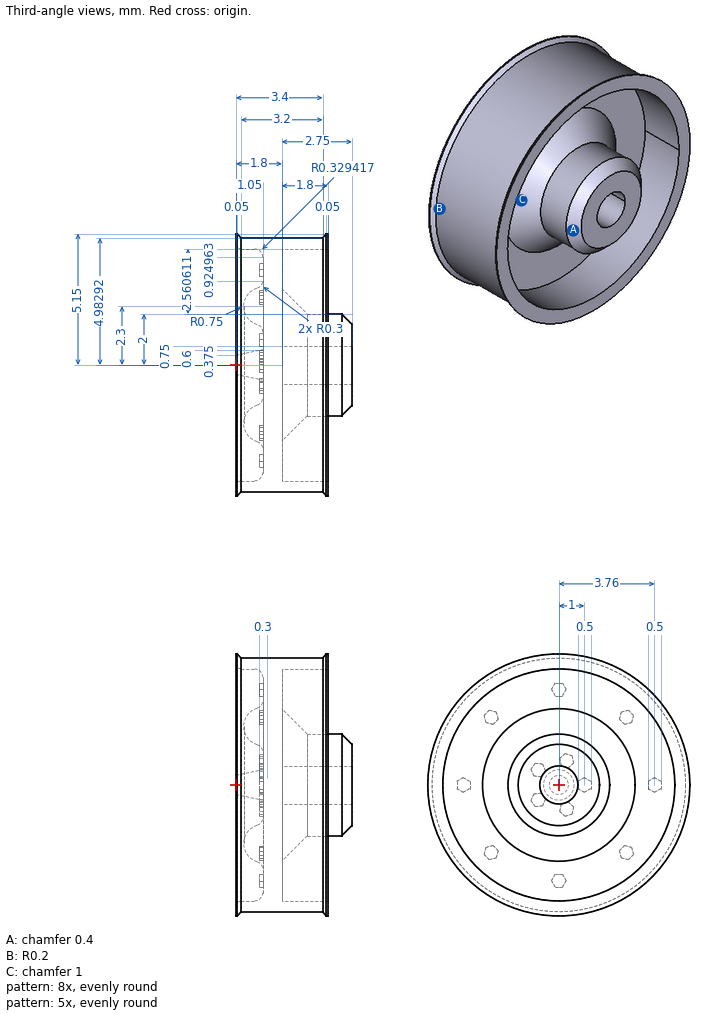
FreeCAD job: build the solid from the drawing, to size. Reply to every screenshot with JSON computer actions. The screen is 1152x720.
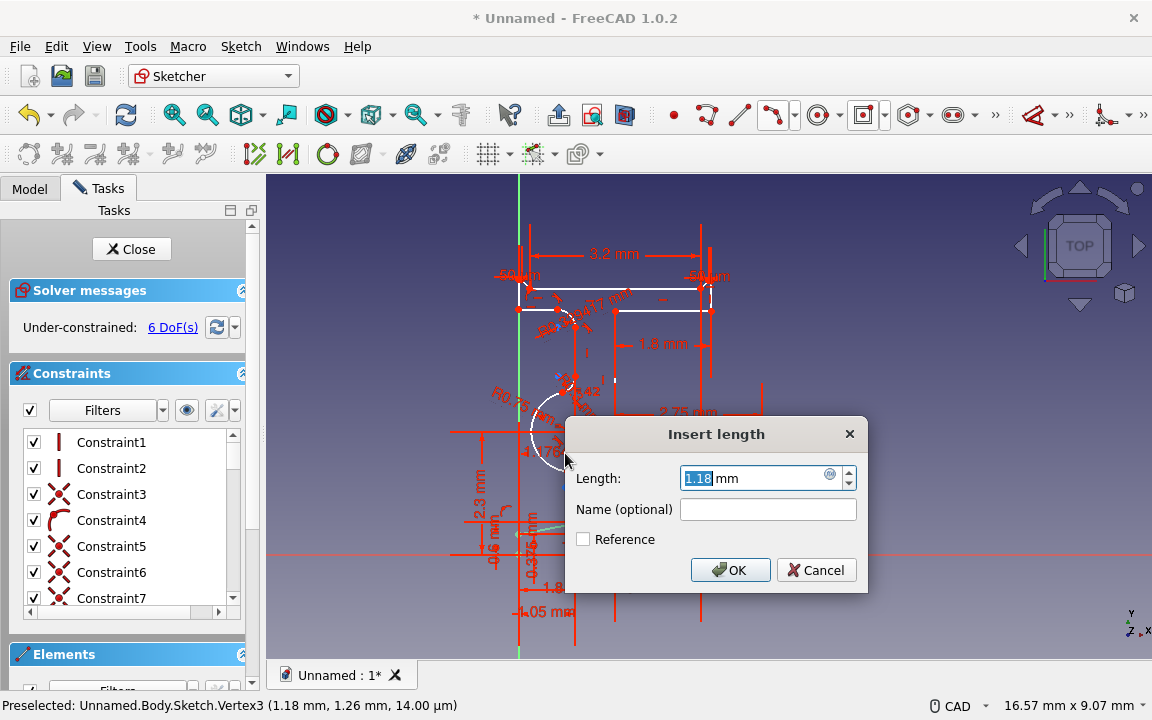
{"action": "type", "text": "1.05"}
{"action": "key", "text": "Return"}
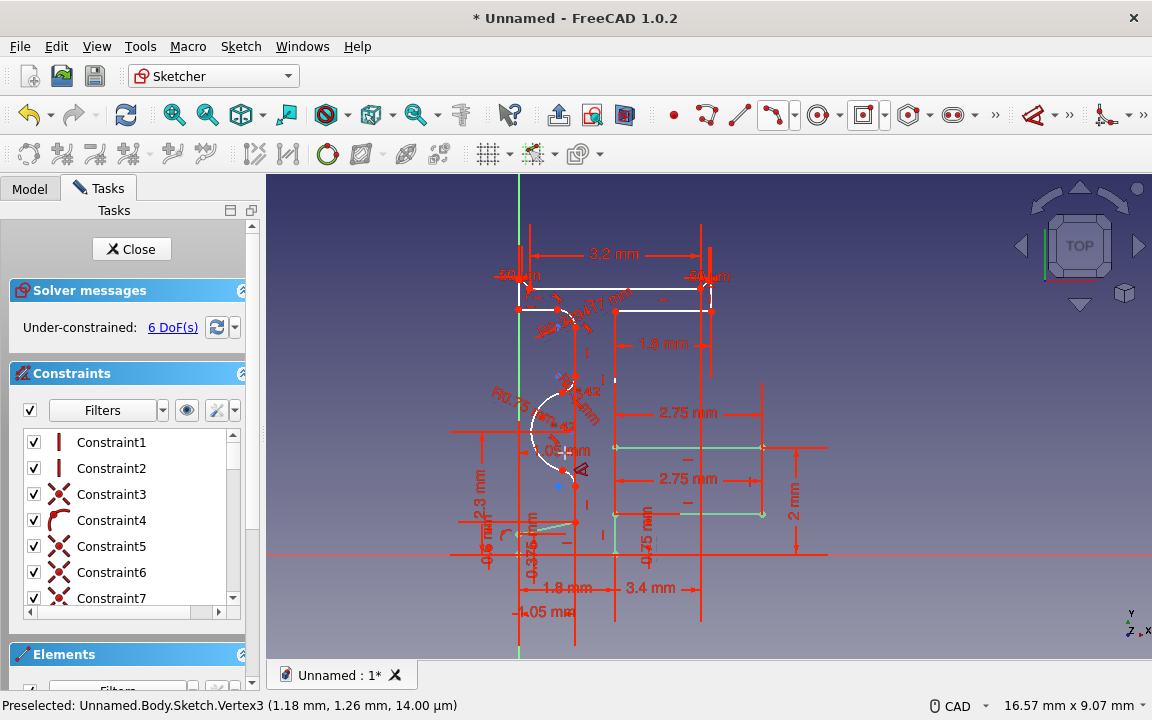
{"action": "scroll", "coordinate": [711, 280], "scroll_direction": "up", "scroll_amount": 8}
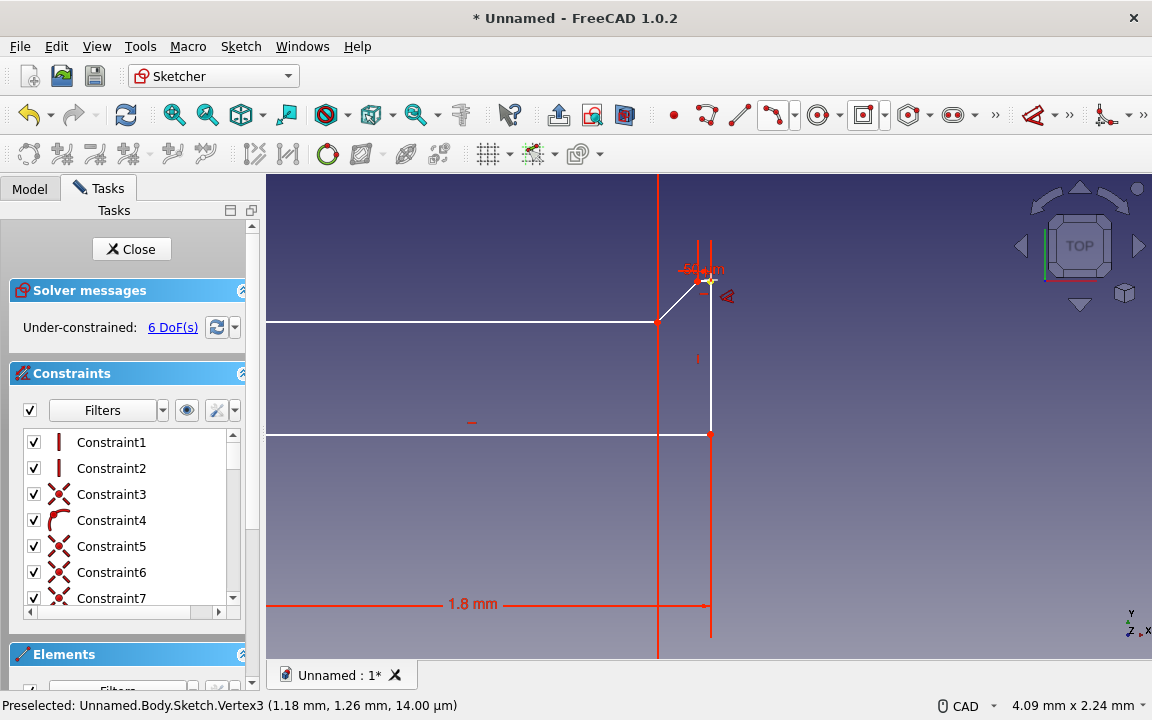
{"action": "left_click", "coordinate": [711, 281]}
{"action": "left_click", "coordinate": [745, 456]}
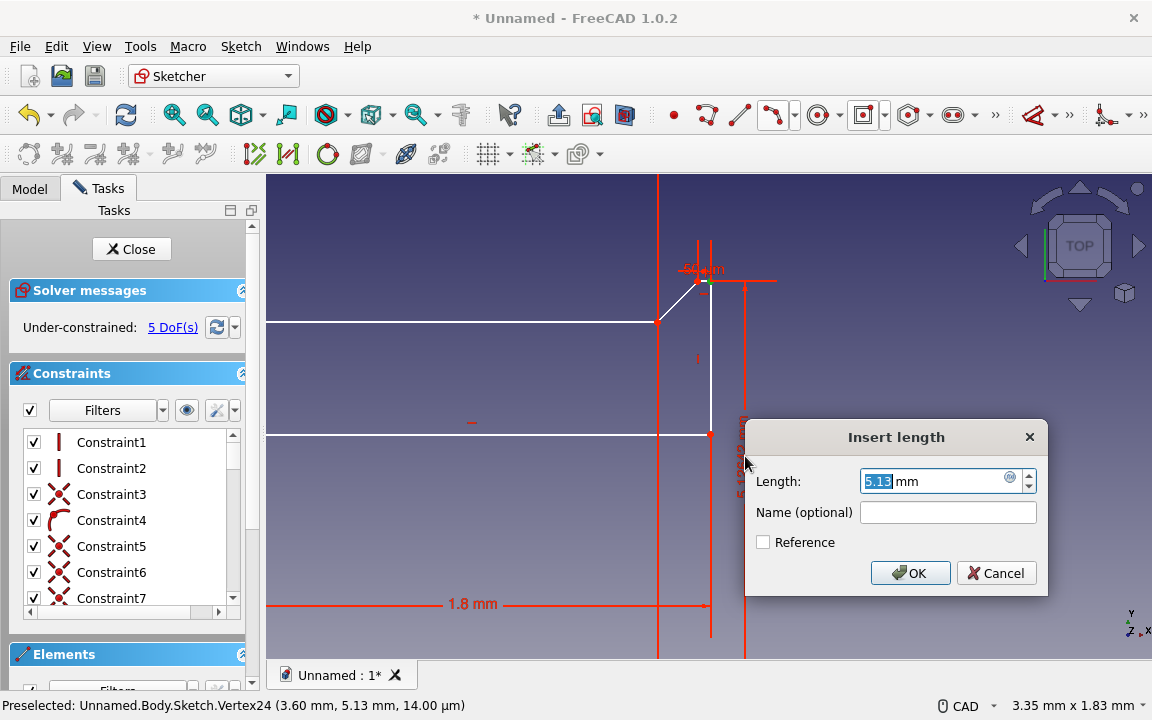
{"action": "type", "text": "5.15"}
{"action": "key", "text": "Return"}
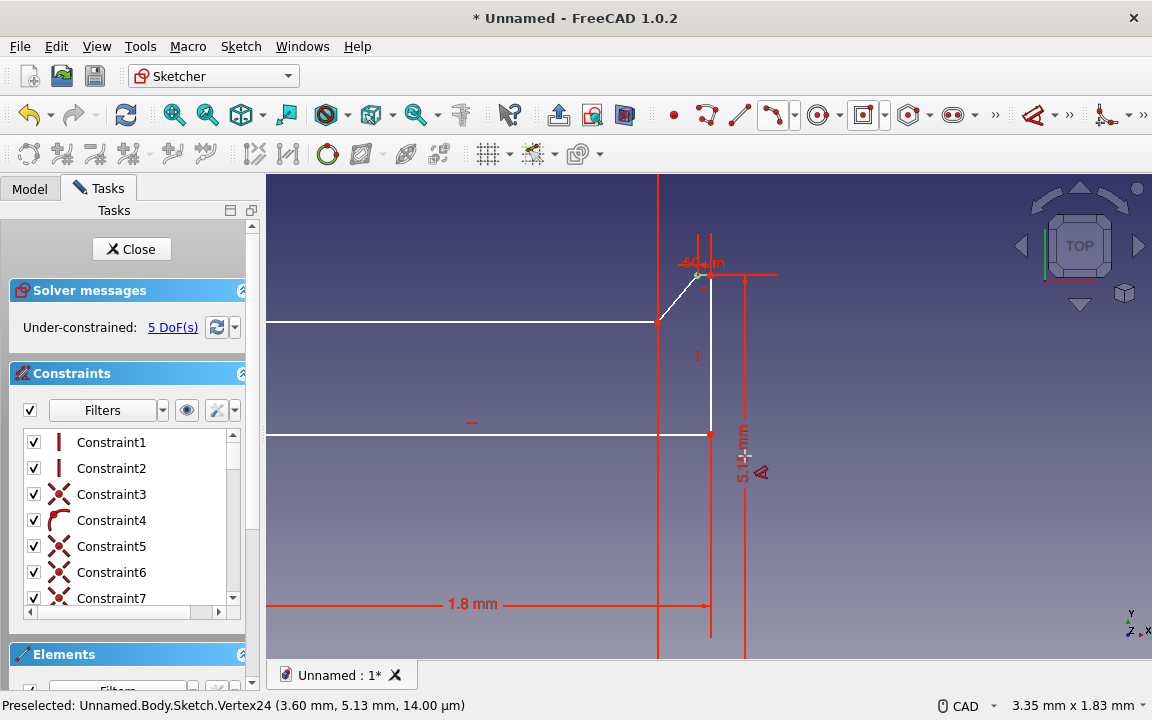
{"action": "scroll", "coordinate": [711, 280], "scroll_direction": "down", "scroll_amount": 8}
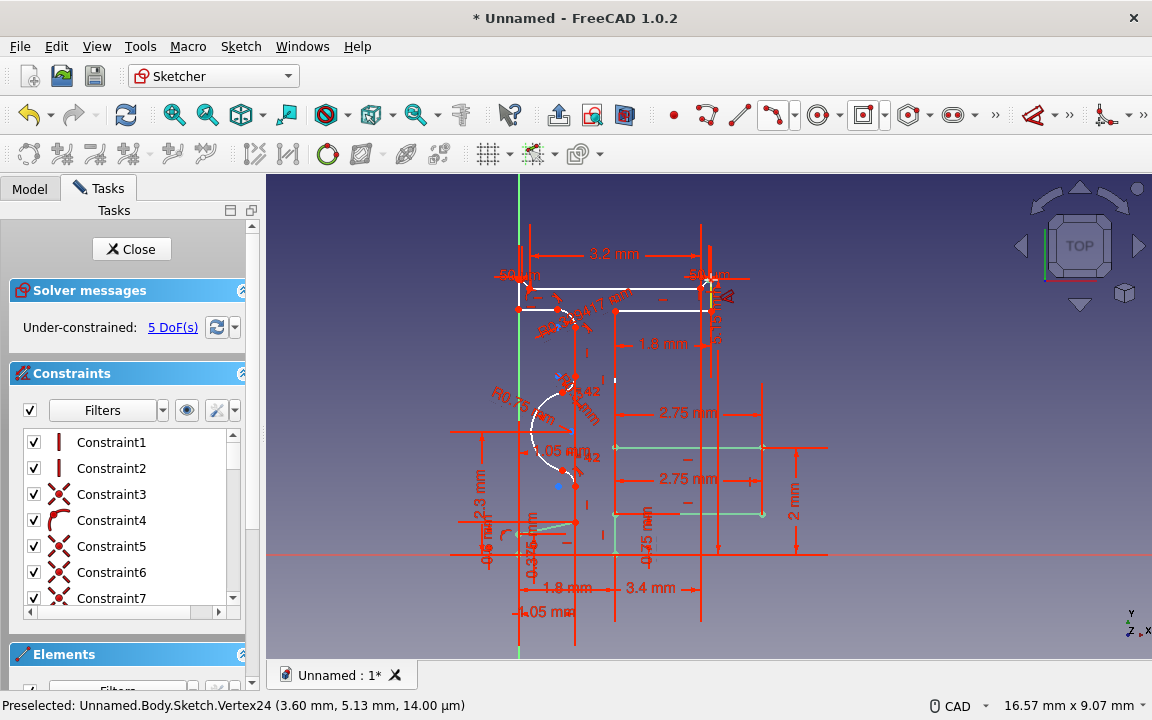
{"action": "scroll", "coordinate": [522, 279], "scroll_direction": "up", "scroll_amount": 8}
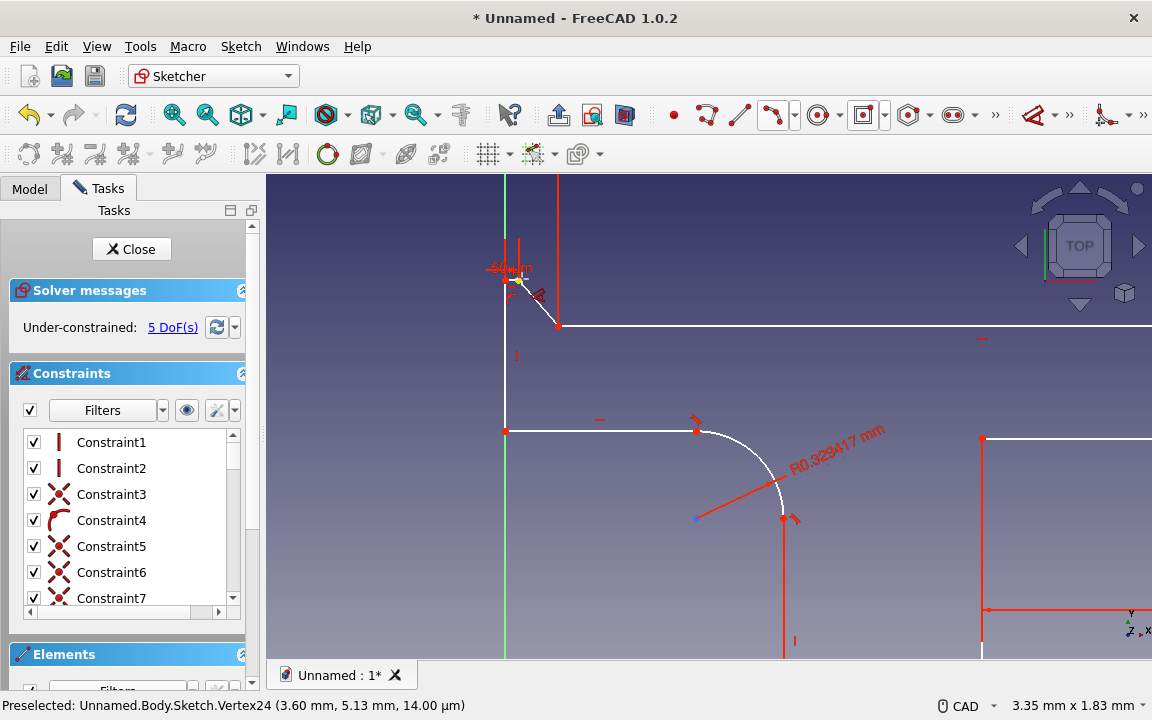
{"action": "left_click", "coordinate": [519, 280]}
{"action": "left_click", "coordinate": [471, 456]}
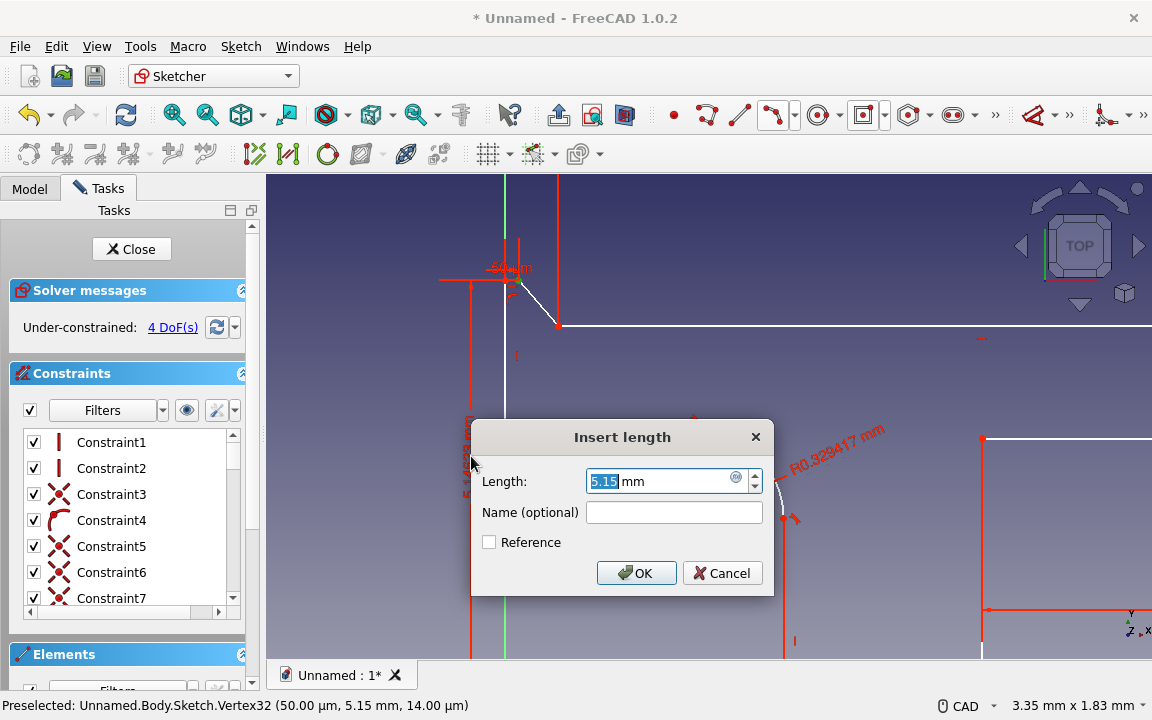
{"action": "type", "text": "5.15"}
{"action": "key", "text": "Return"}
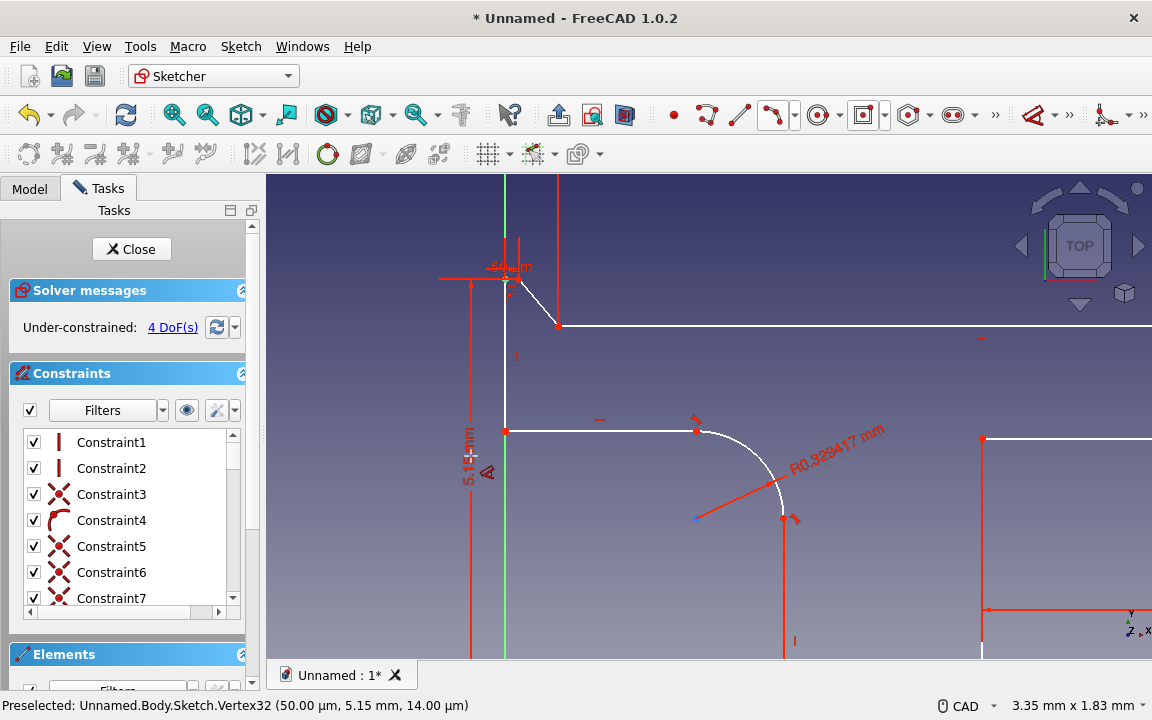
{"action": "scroll", "coordinate": [522, 279], "scroll_direction": "down", "scroll_amount": 8}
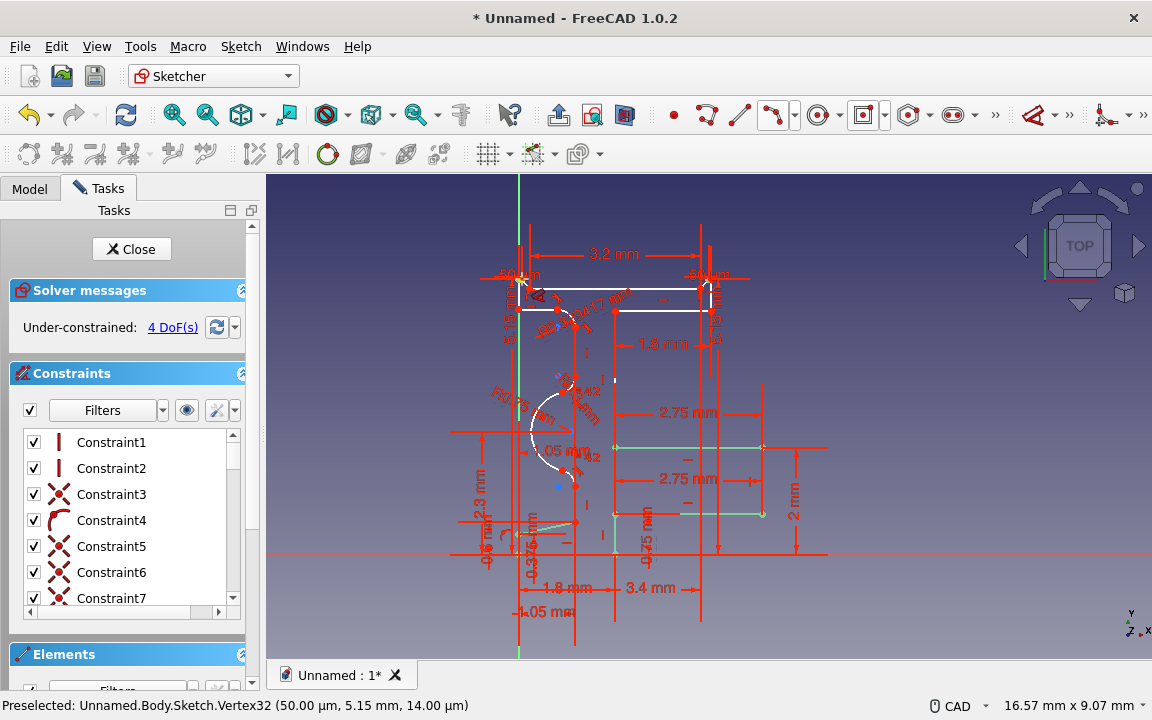
{"action": "left_click", "coordinate": [571, 432]}
{"action": "left_click", "coordinate": [545, 374]}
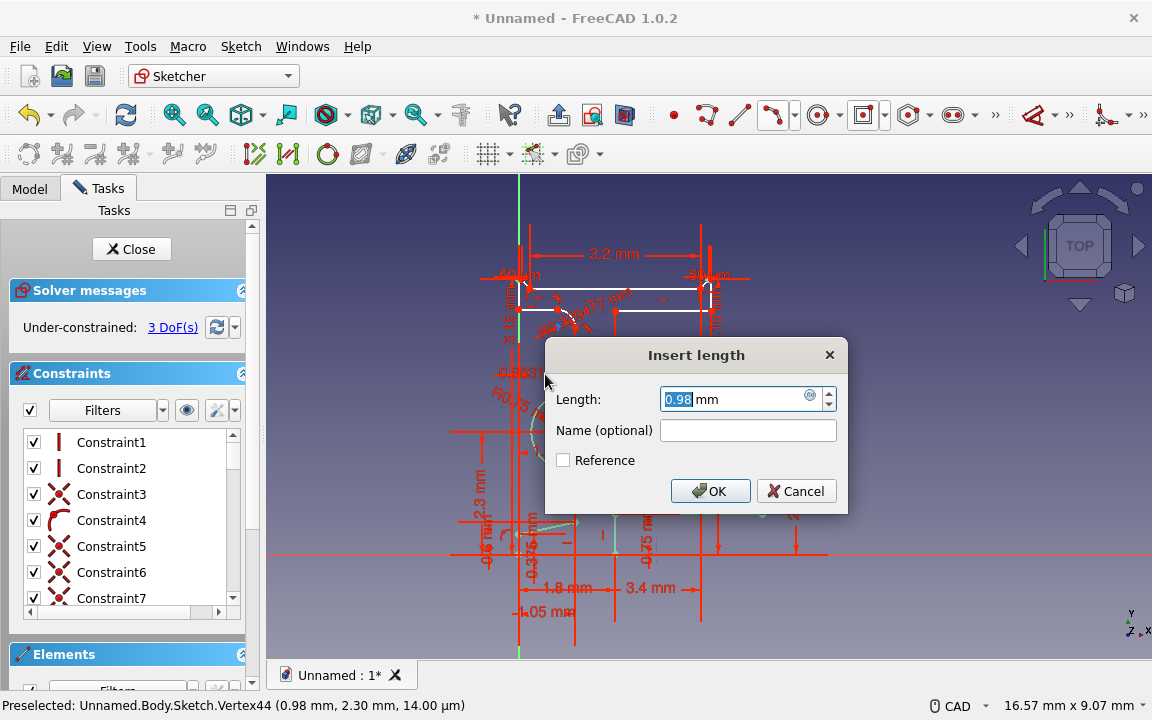
{"action": "type", "text": "1.05"}
{"action": "key", "text": "Return"}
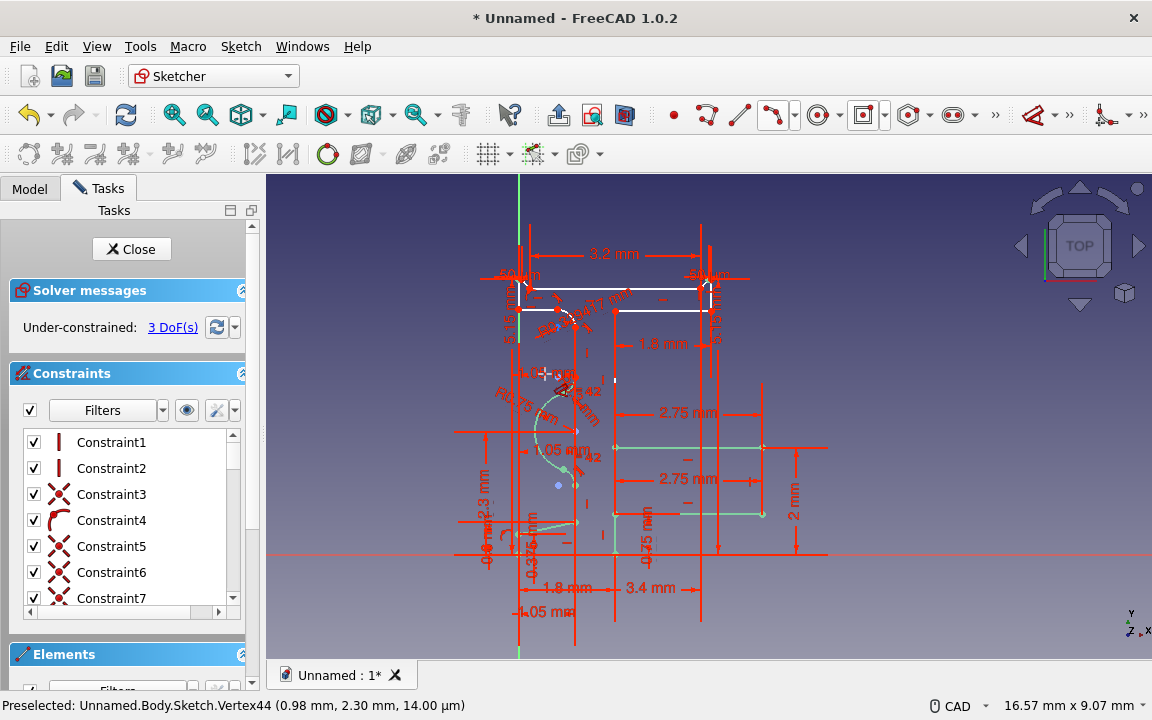
{"action": "left_click", "coordinate": [575, 343]}
{"action": "left_click", "coordinate": [541, 353]}